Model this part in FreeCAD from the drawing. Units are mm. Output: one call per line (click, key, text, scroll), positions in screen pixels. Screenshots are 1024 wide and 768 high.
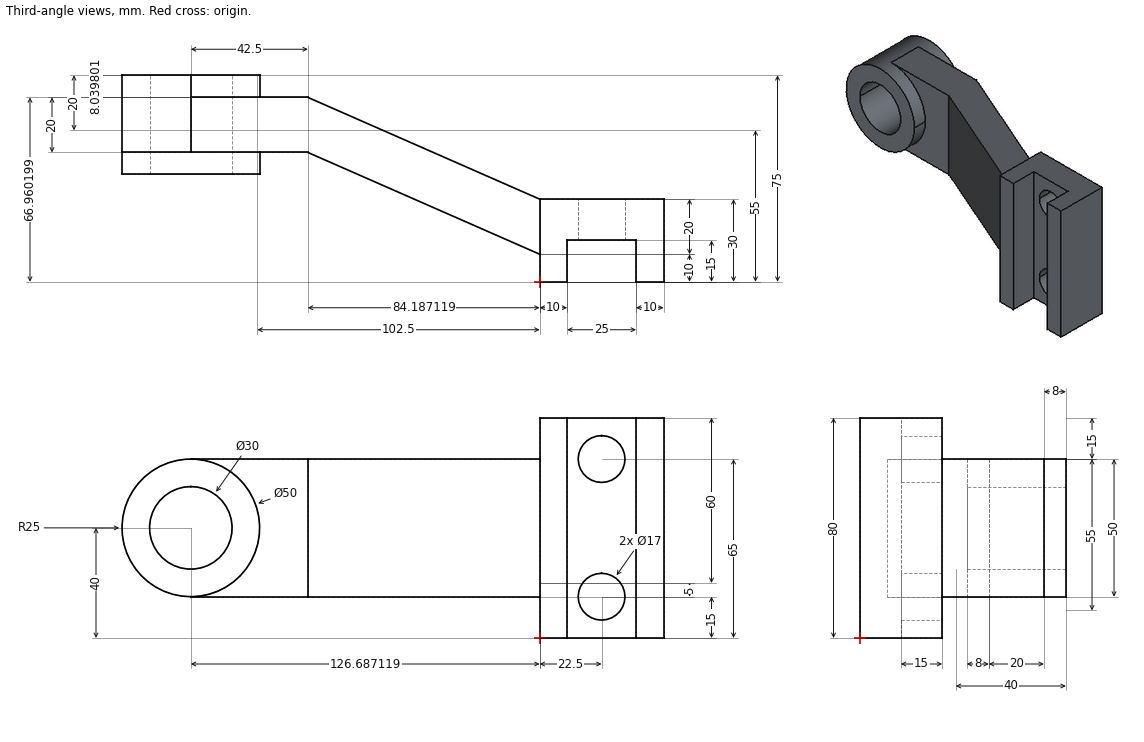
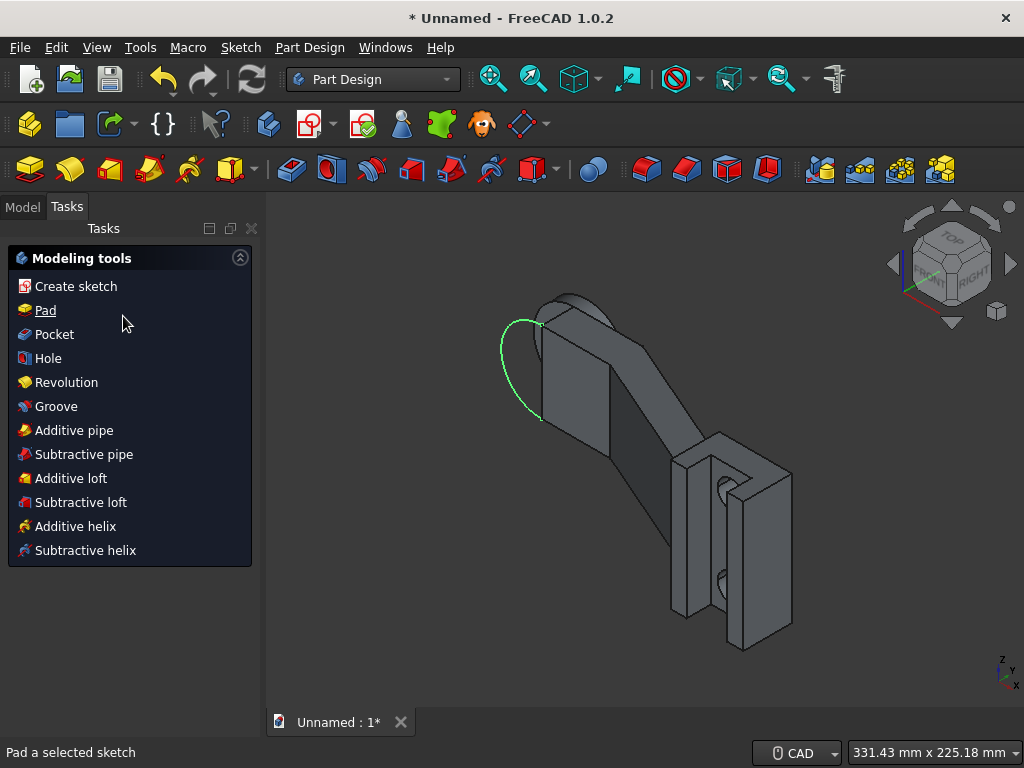
click(30, 170)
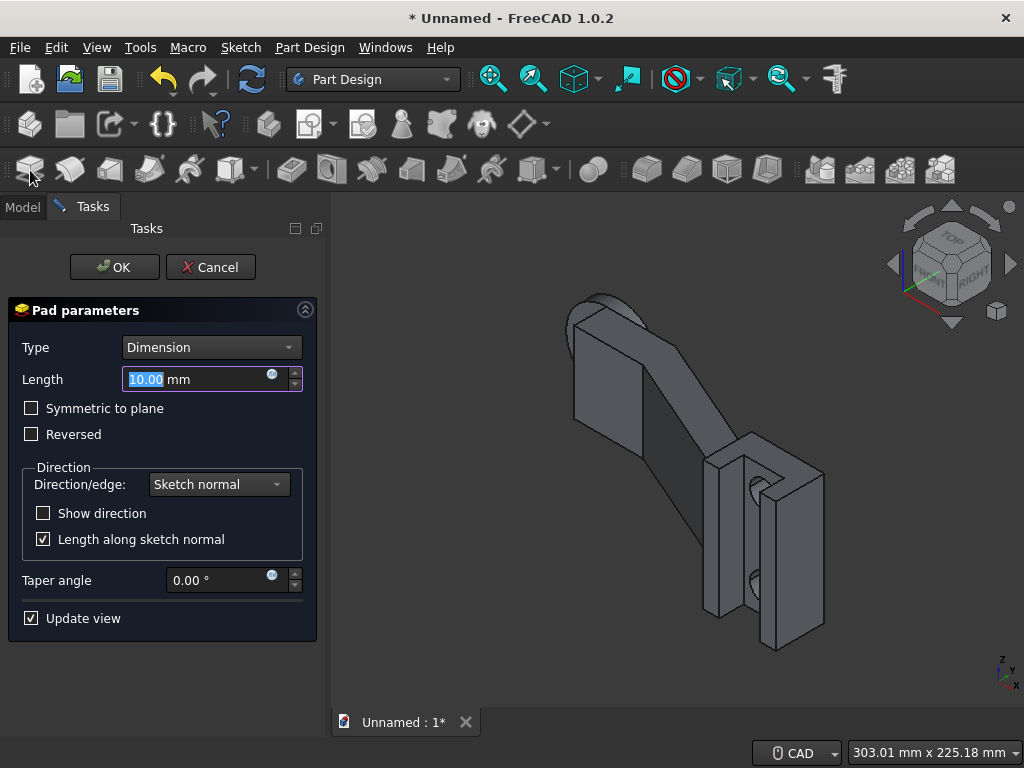
text(20)
key(Tab)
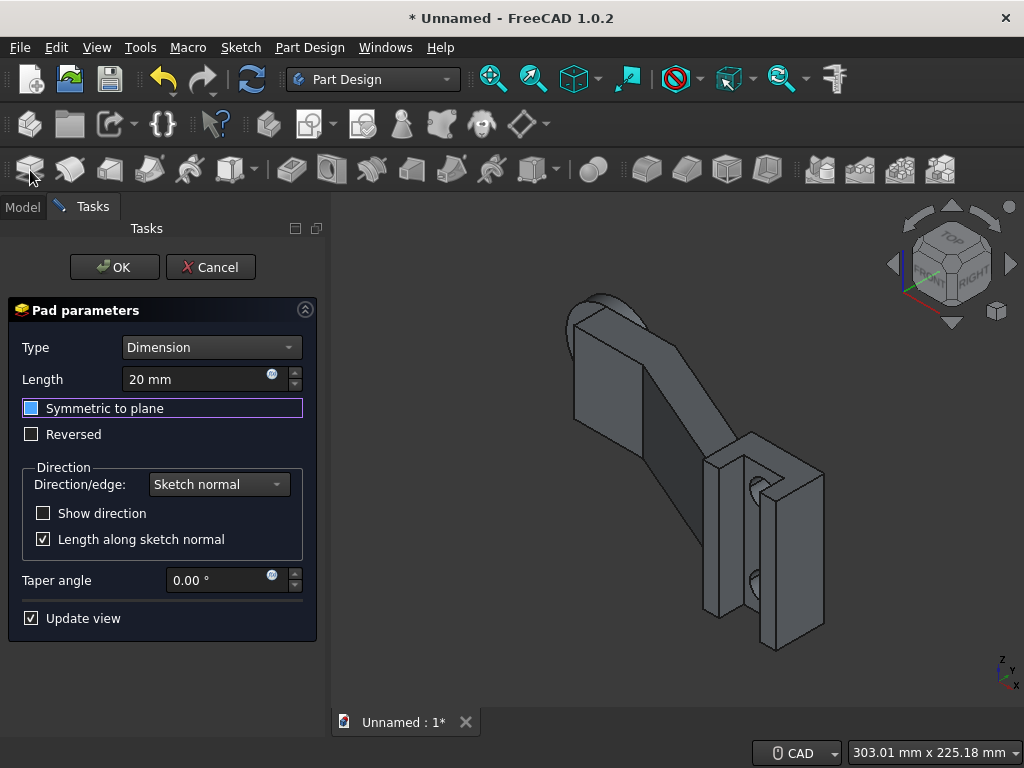
click(30, 434)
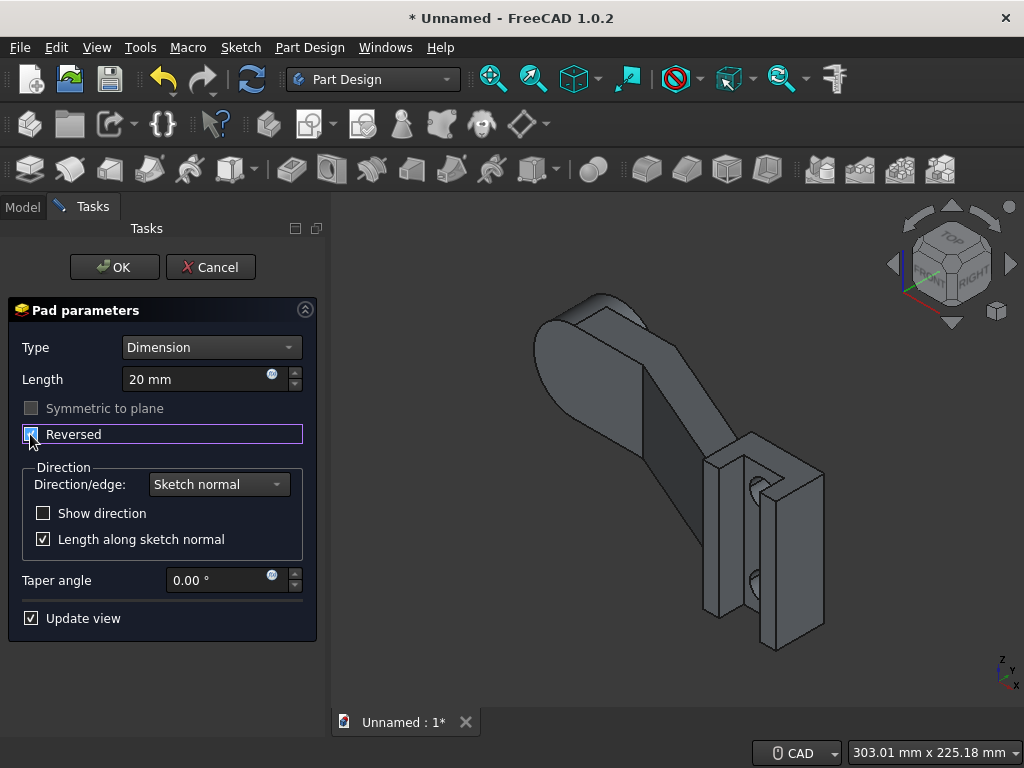
click(115, 267)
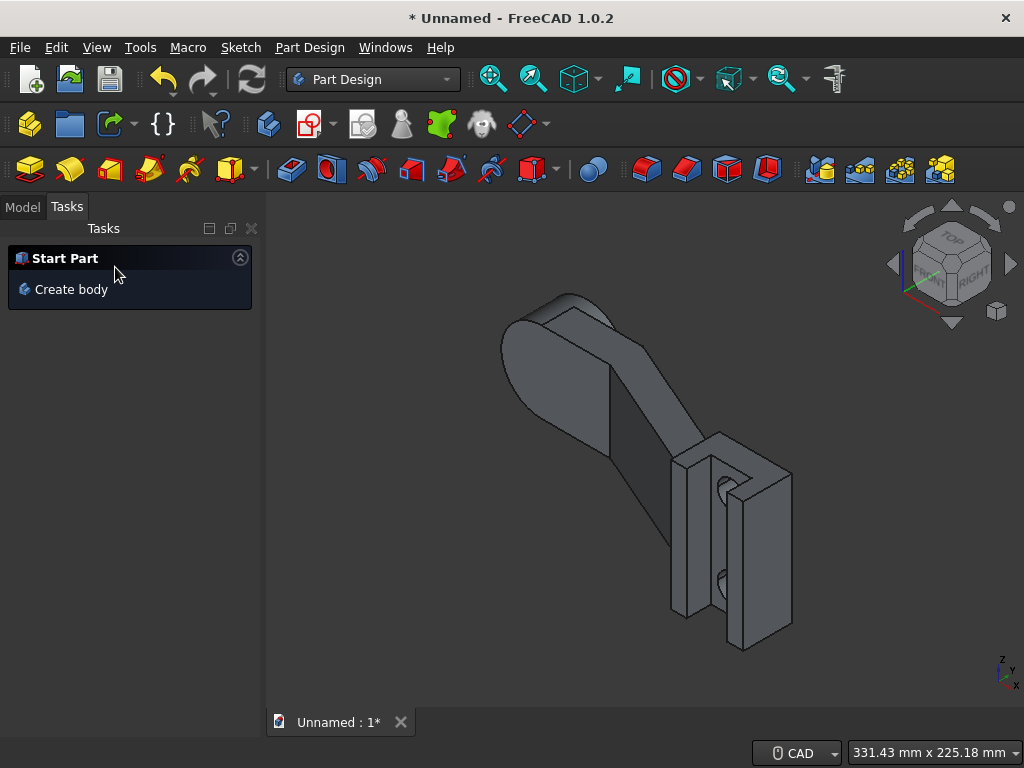
click(23, 206)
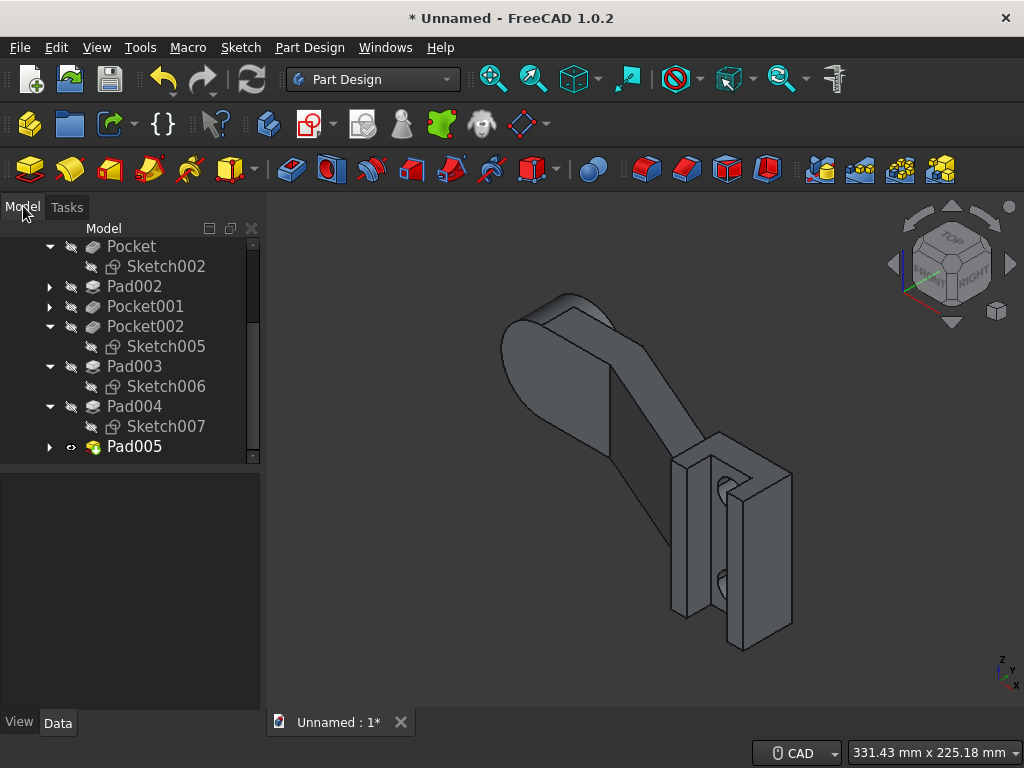
scroll(140, 342, down, 3)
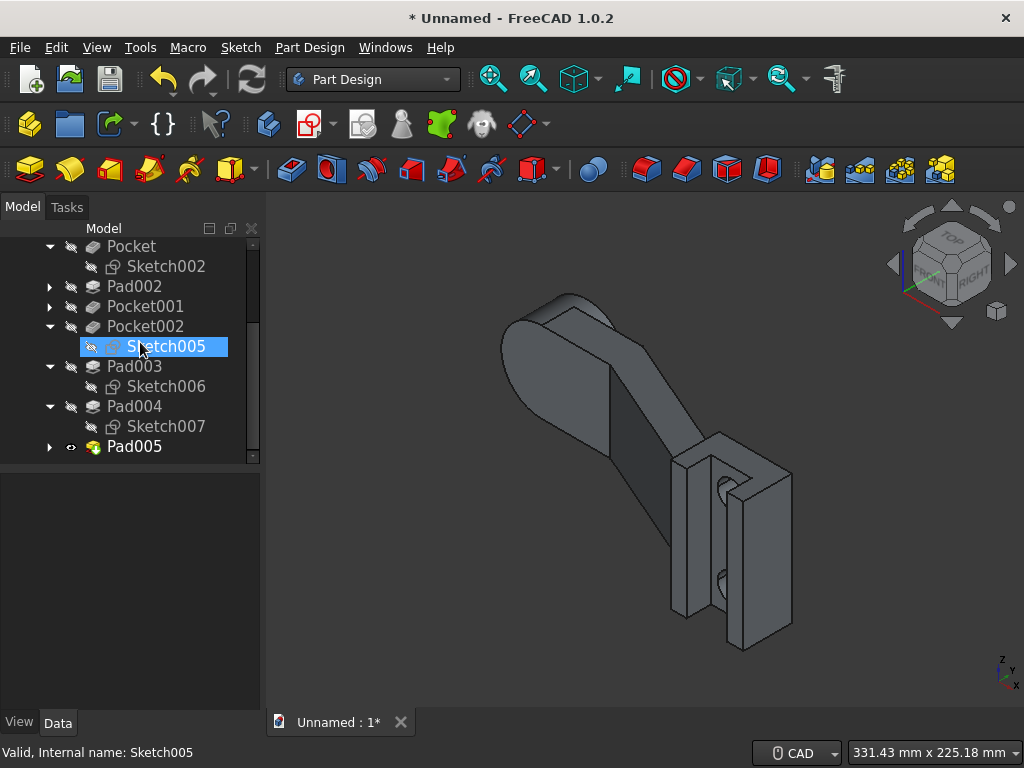
scroll(140, 342, up, 15)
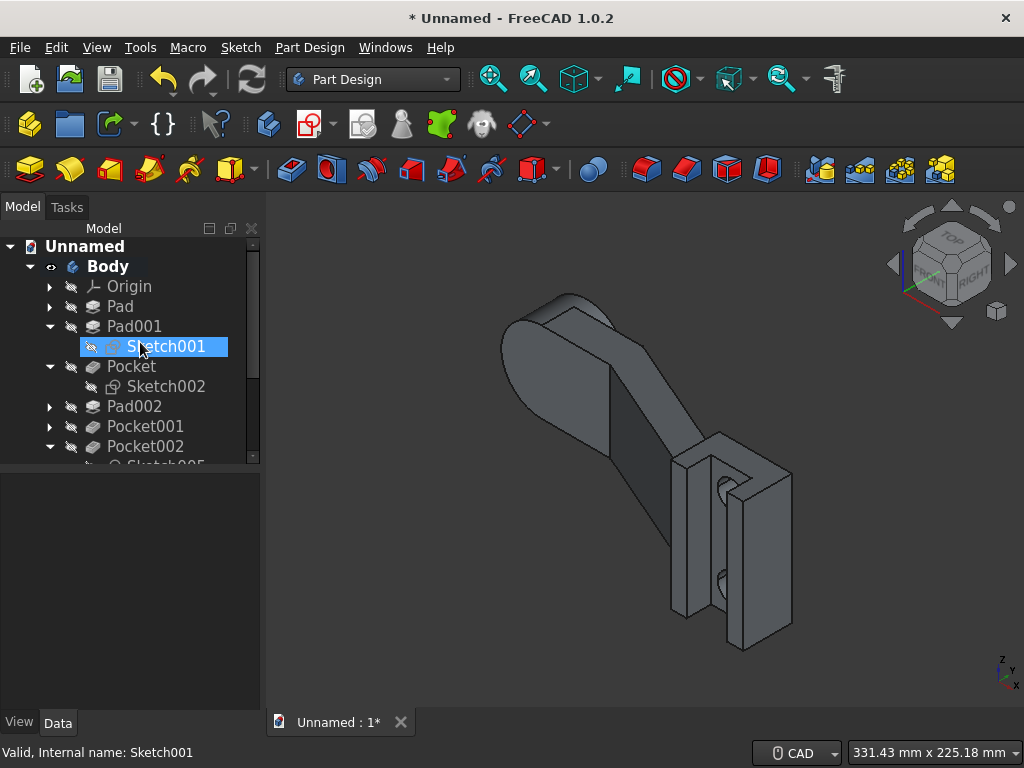
click(50, 287)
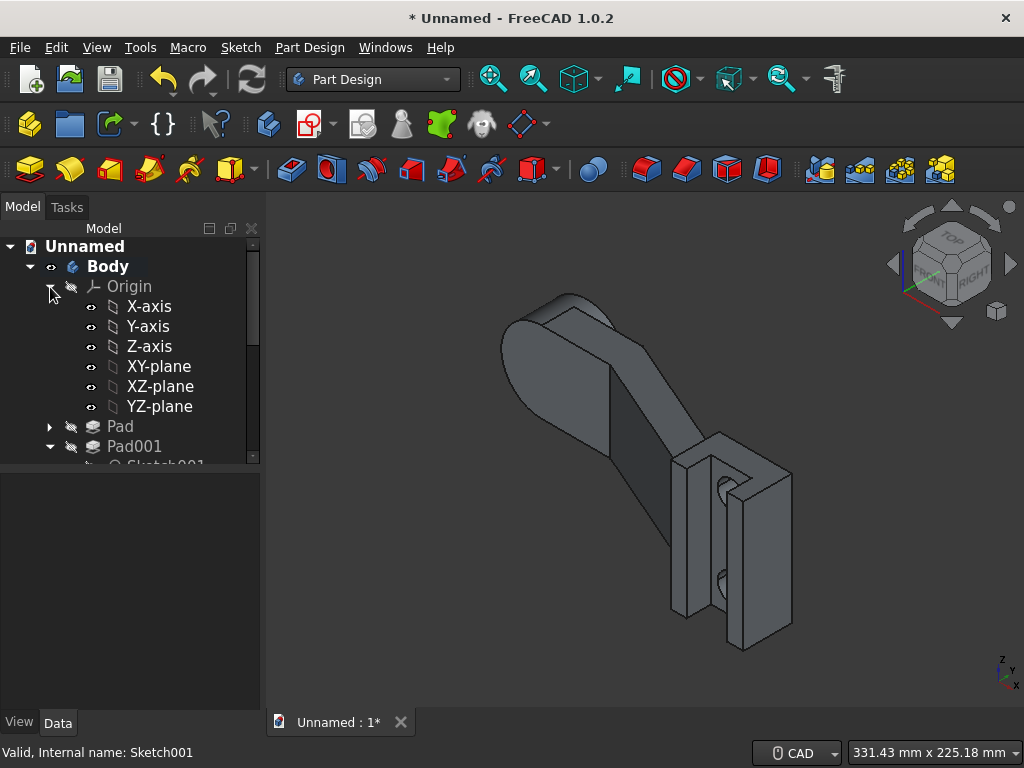
click(136, 387)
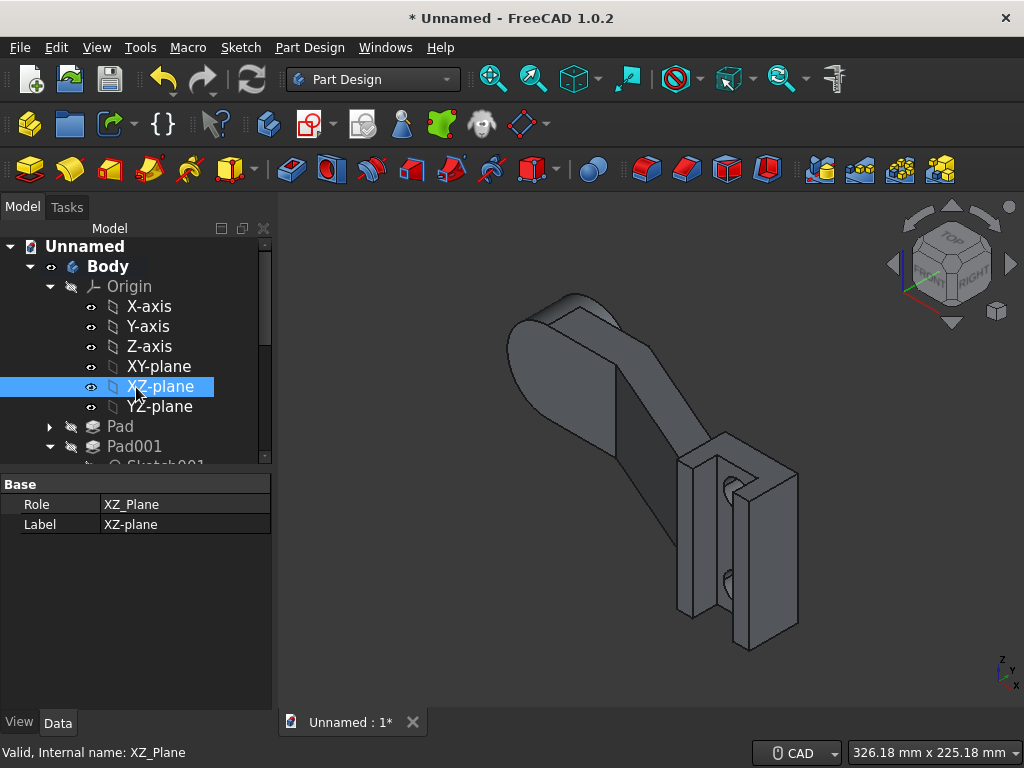
click(522, 124)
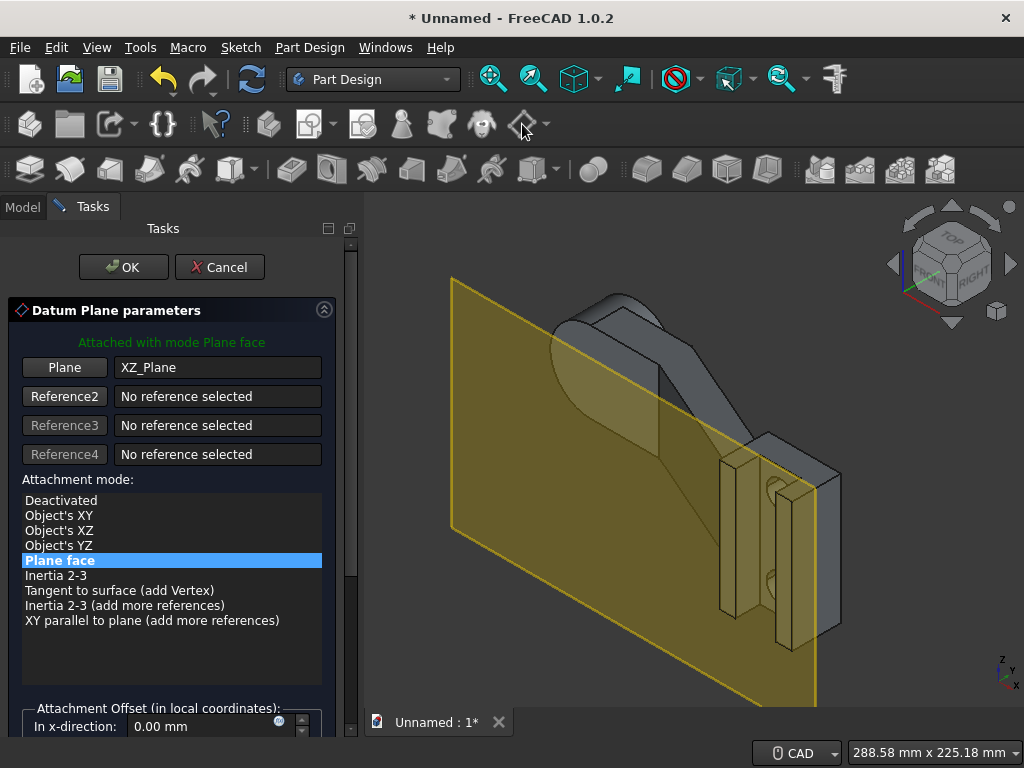
scroll(351, 487, down, 3)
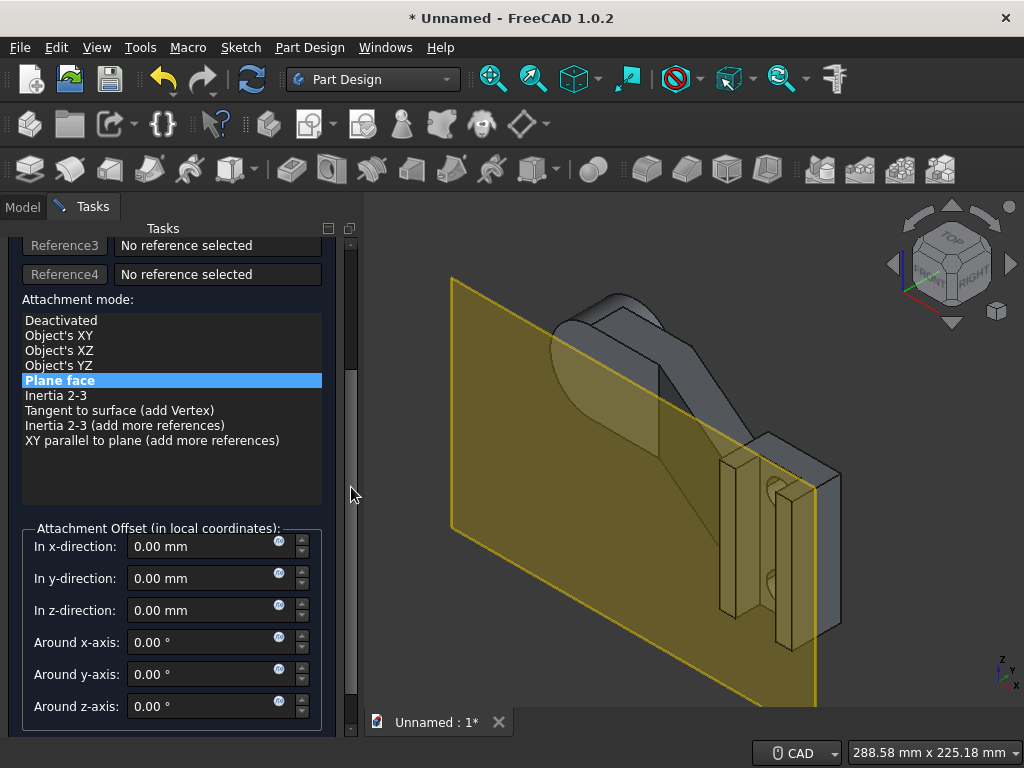
triple_click(210, 610)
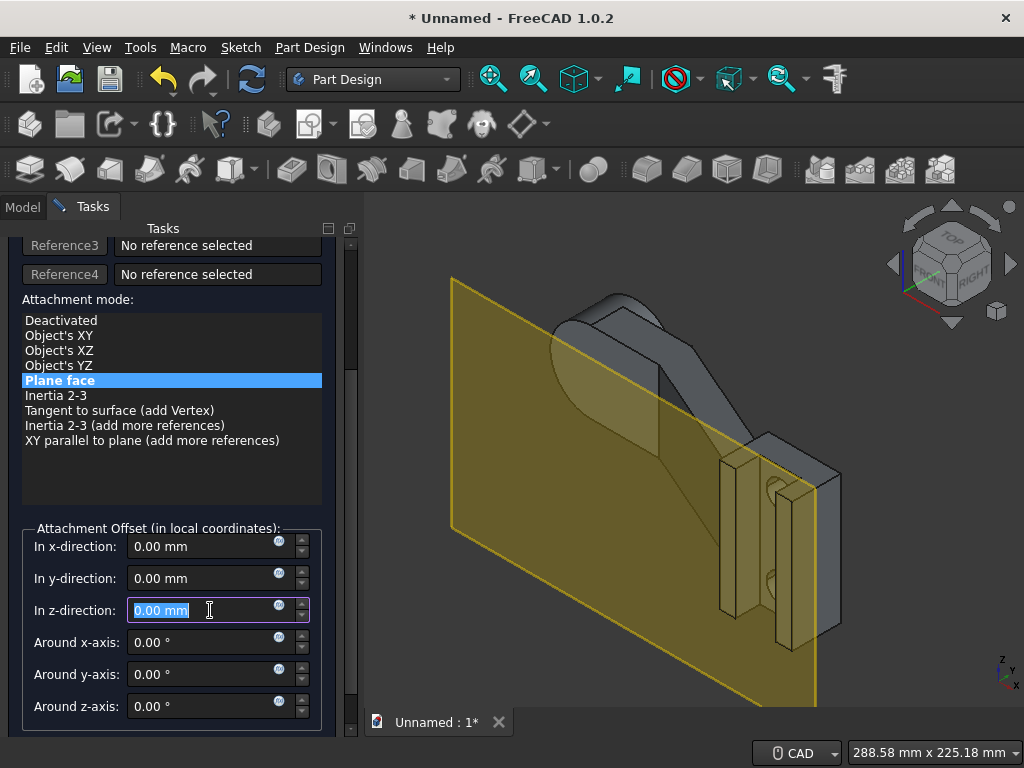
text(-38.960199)
key(Tab)